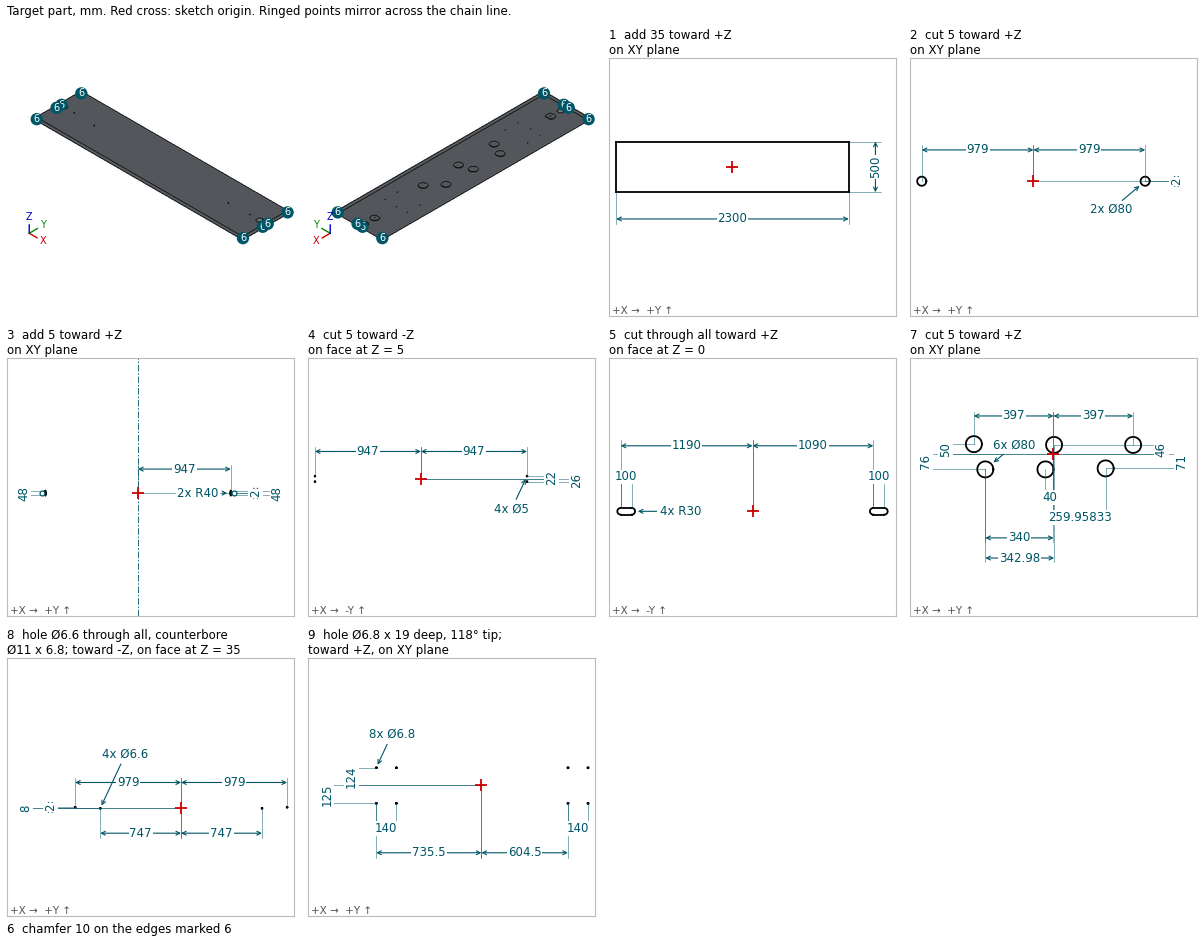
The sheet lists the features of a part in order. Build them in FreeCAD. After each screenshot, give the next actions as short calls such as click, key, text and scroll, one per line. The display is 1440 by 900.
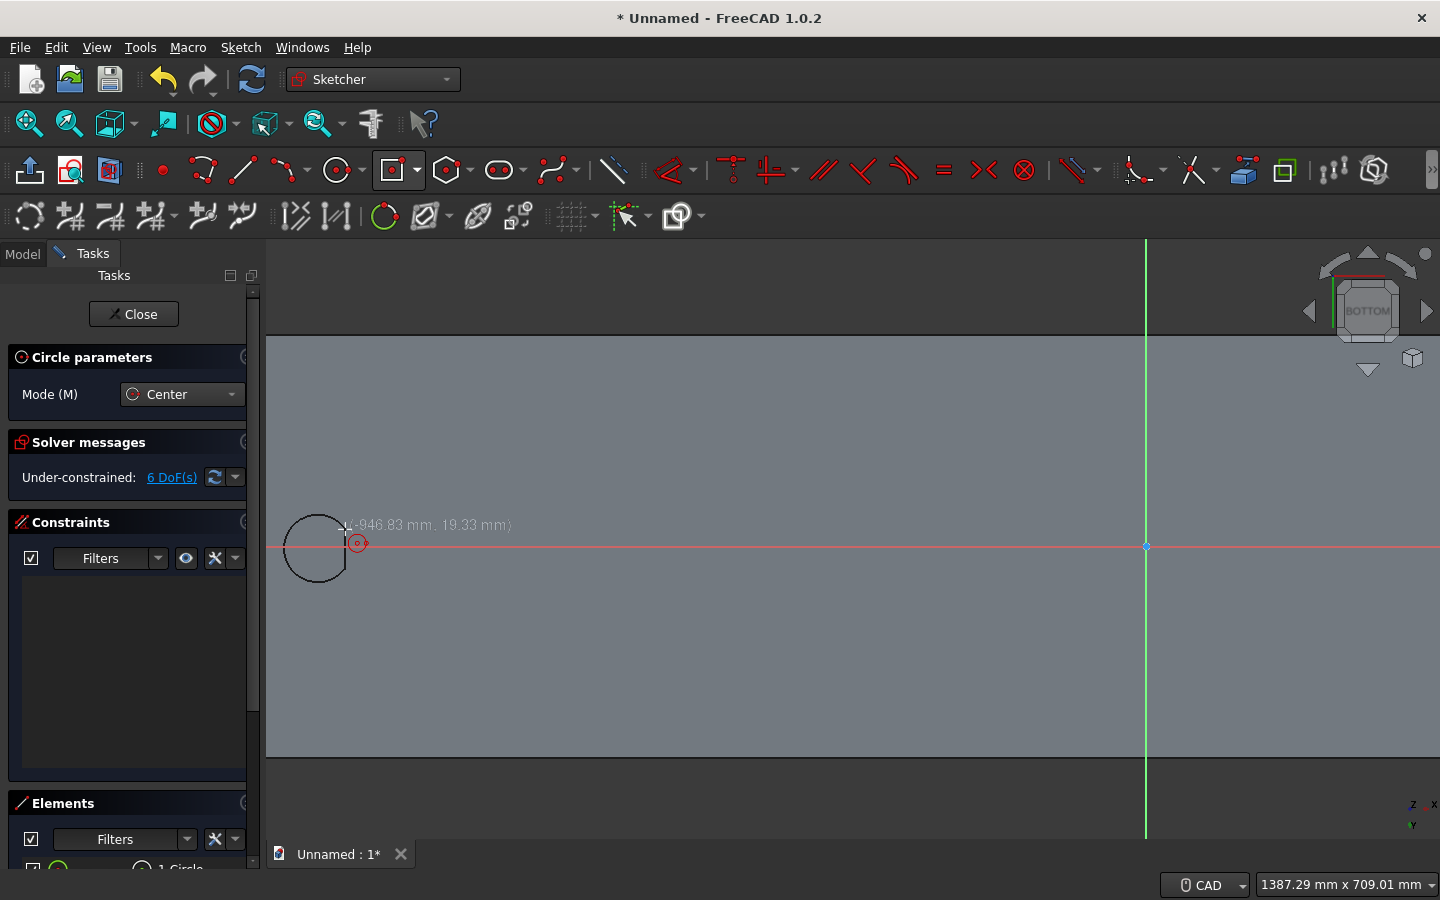
click(345, 528)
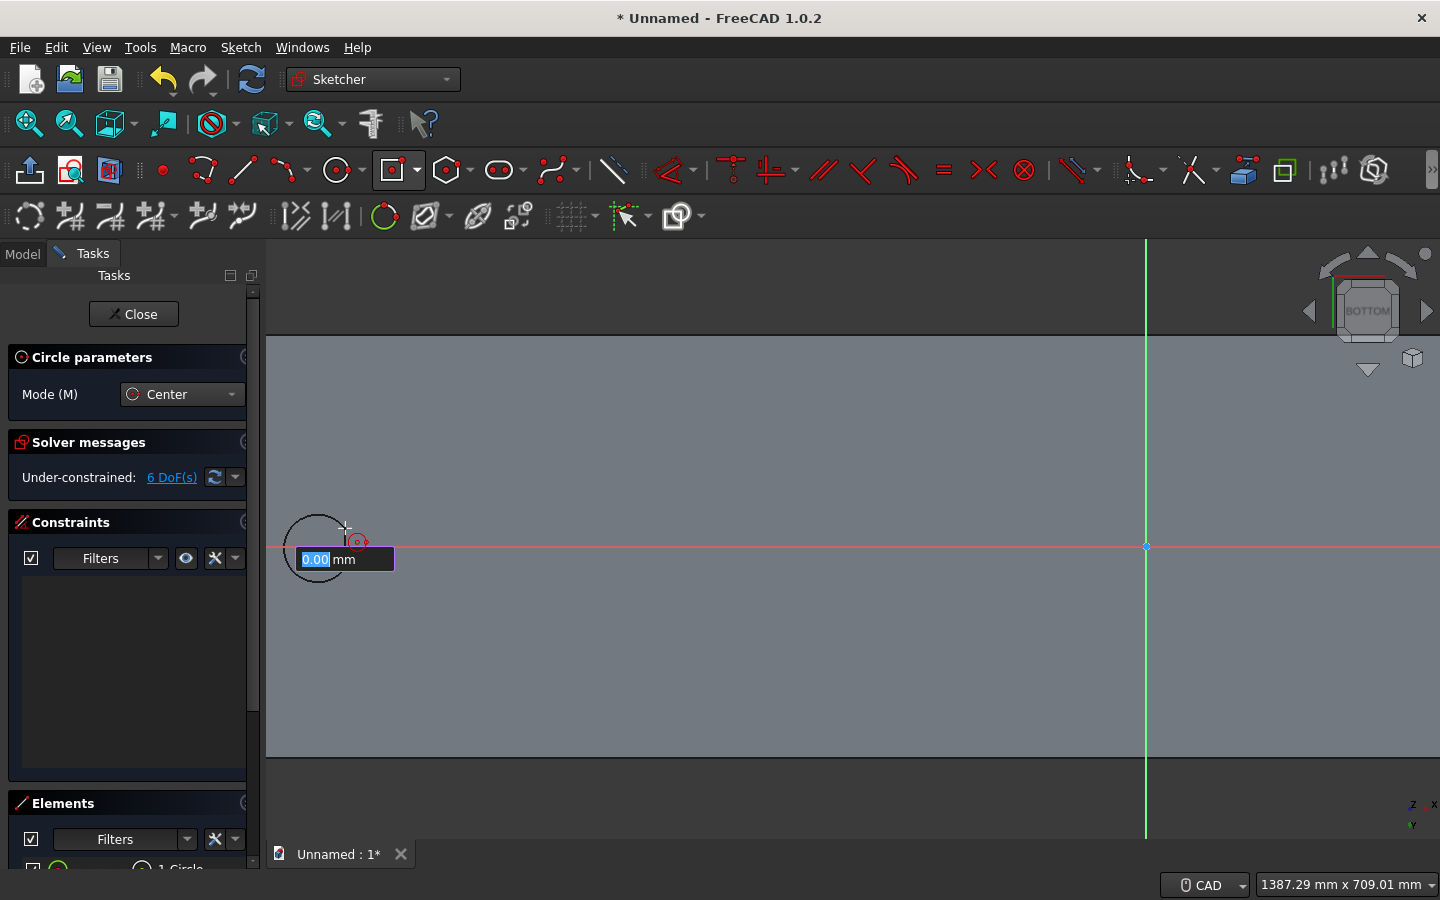
scroll(346, 527, up, 11)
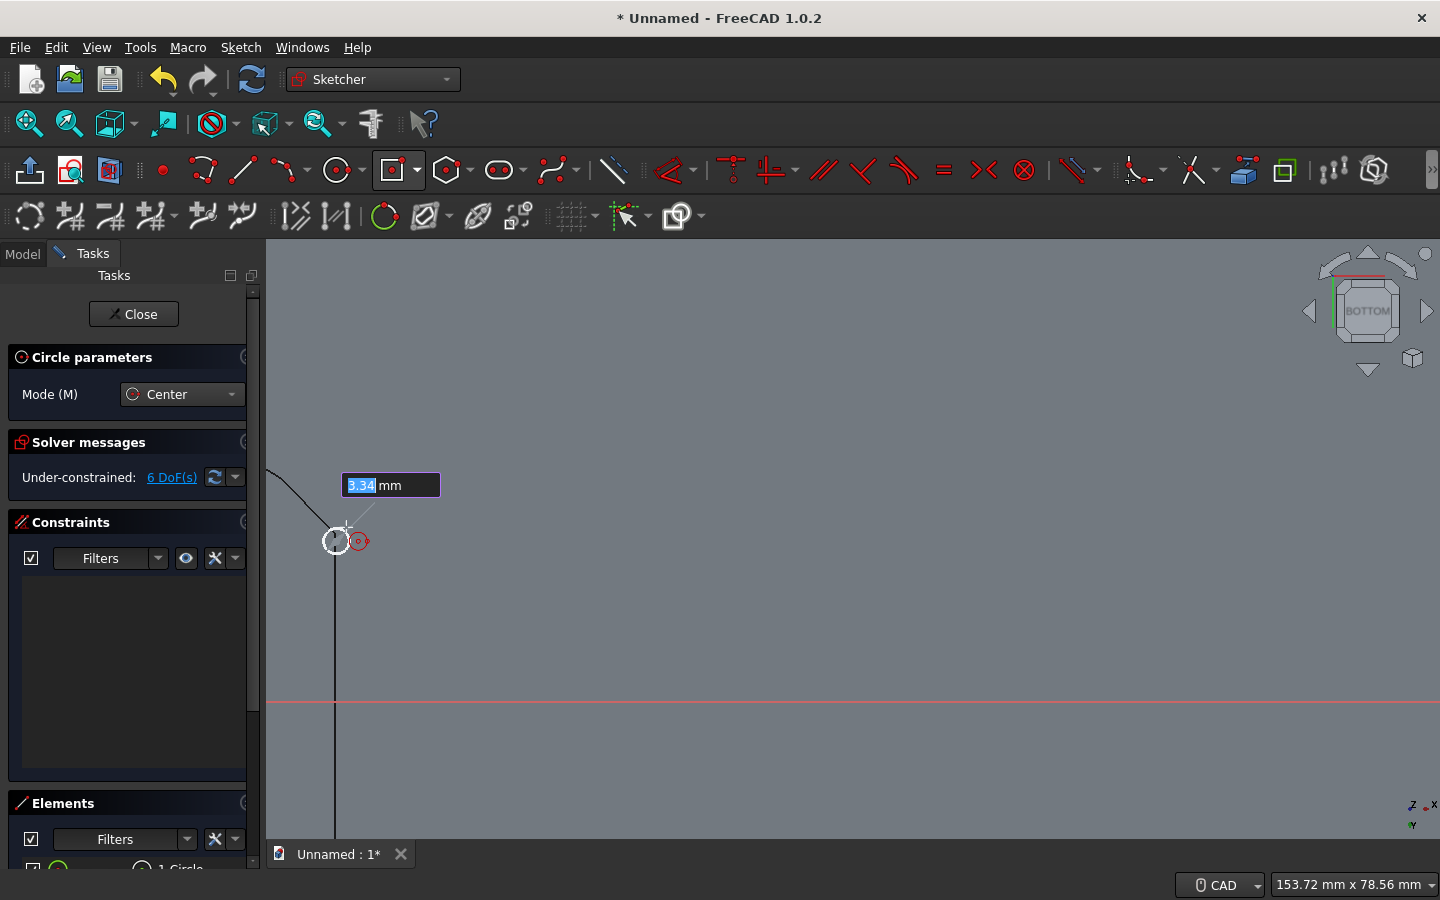
click(348, 520)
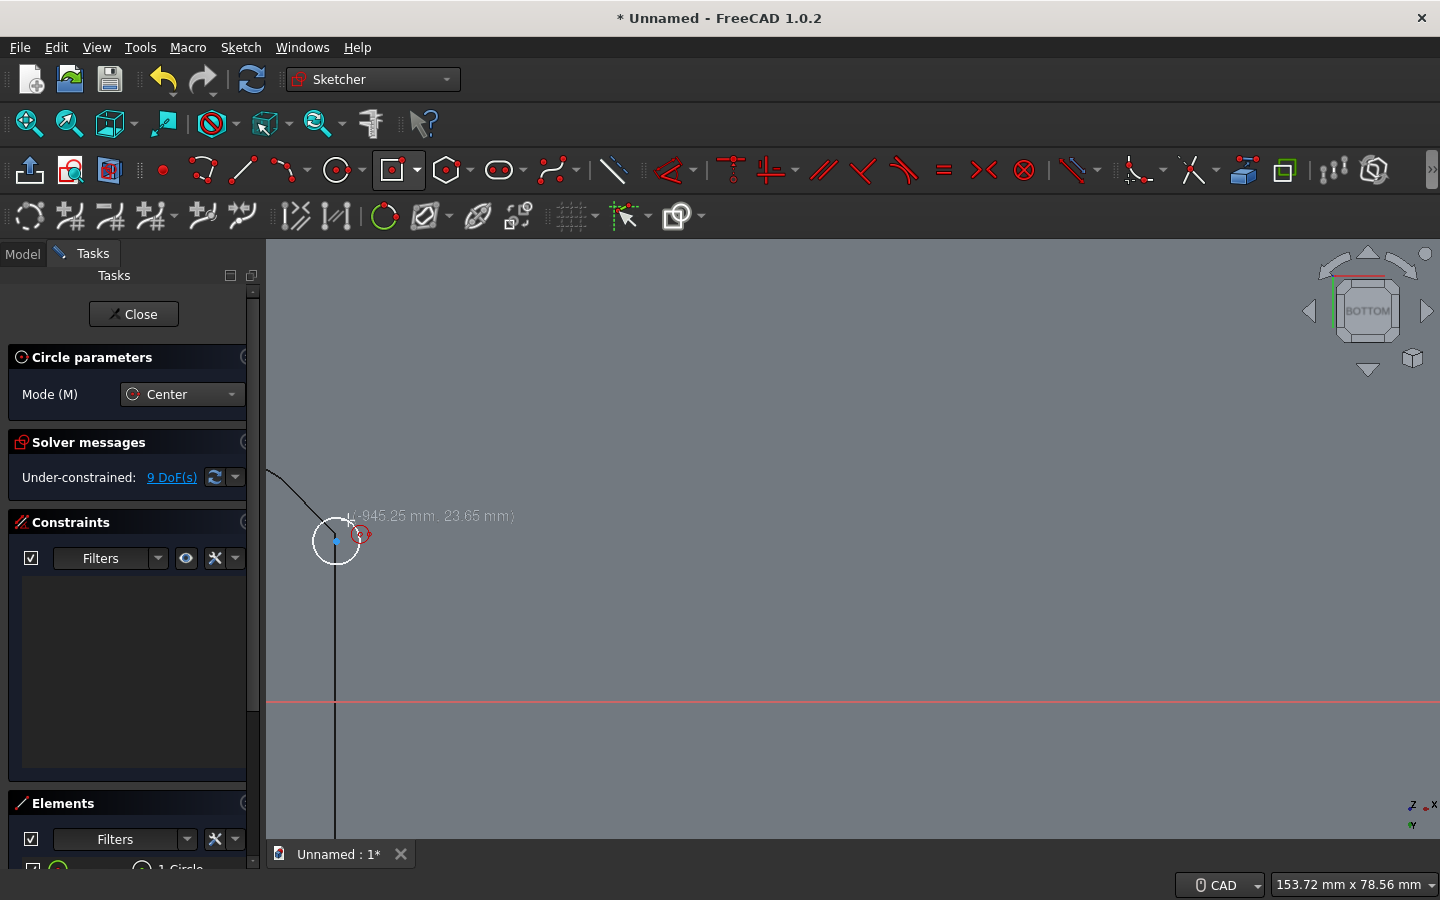
scroll(429, 530, down, 15)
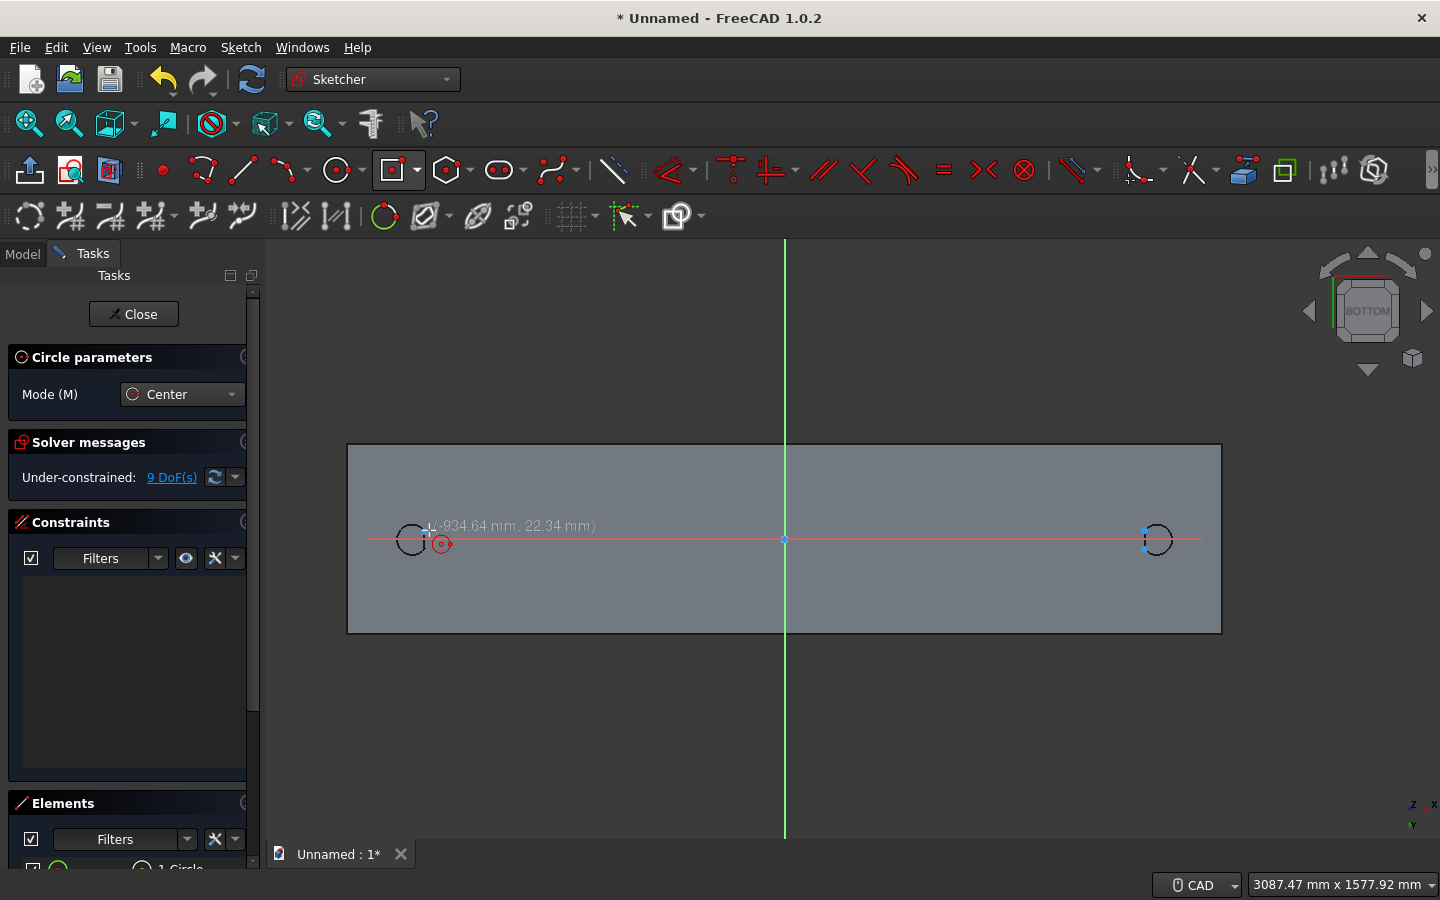
scroll(424, 549, up, 16)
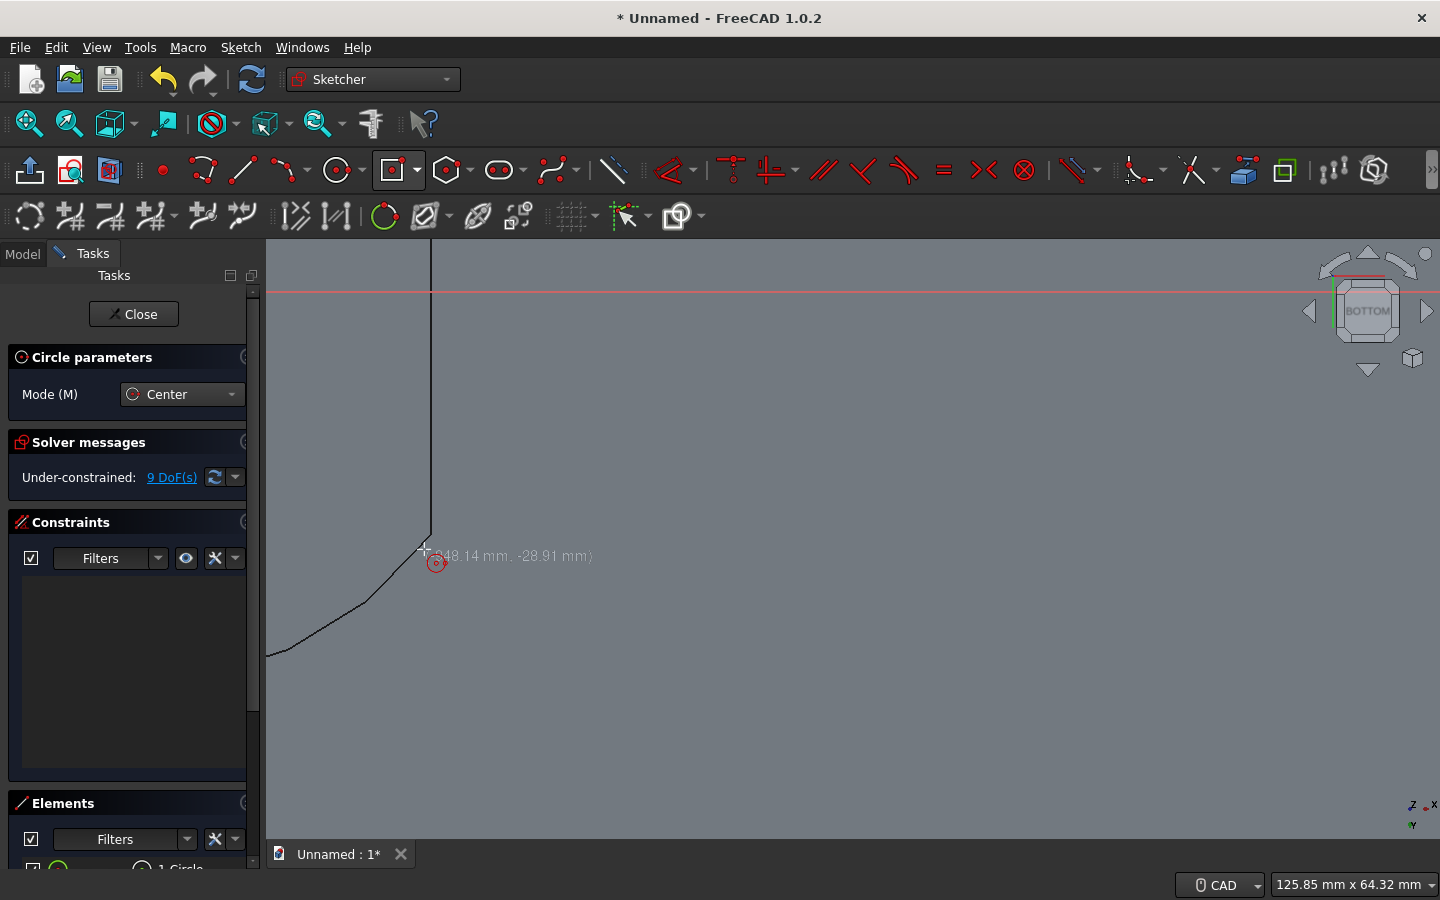
scroll(340, 551, down, 15)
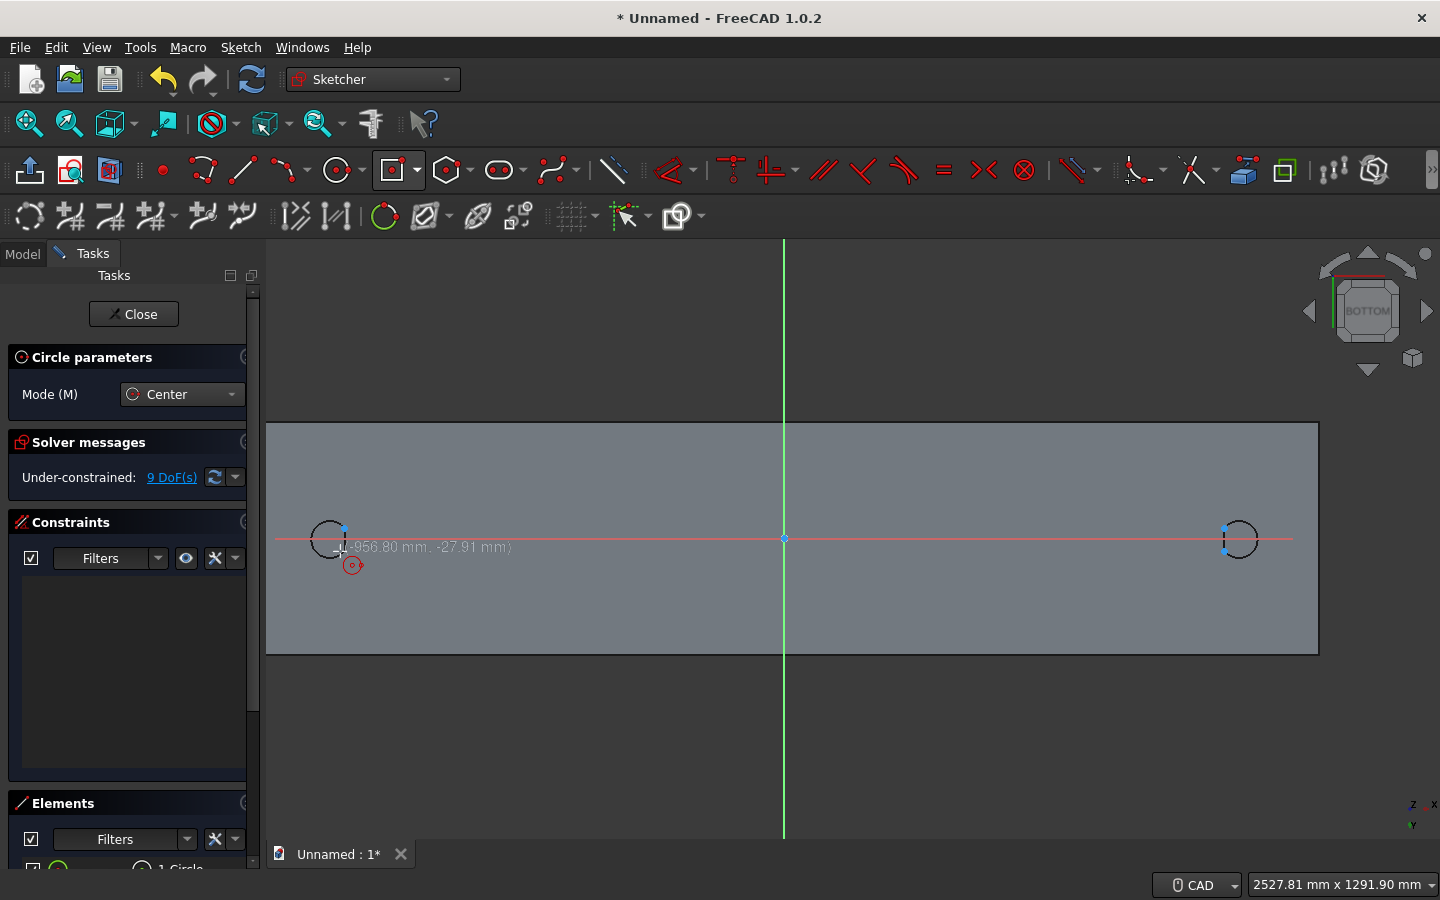
scroll(345, 551, up, 2)